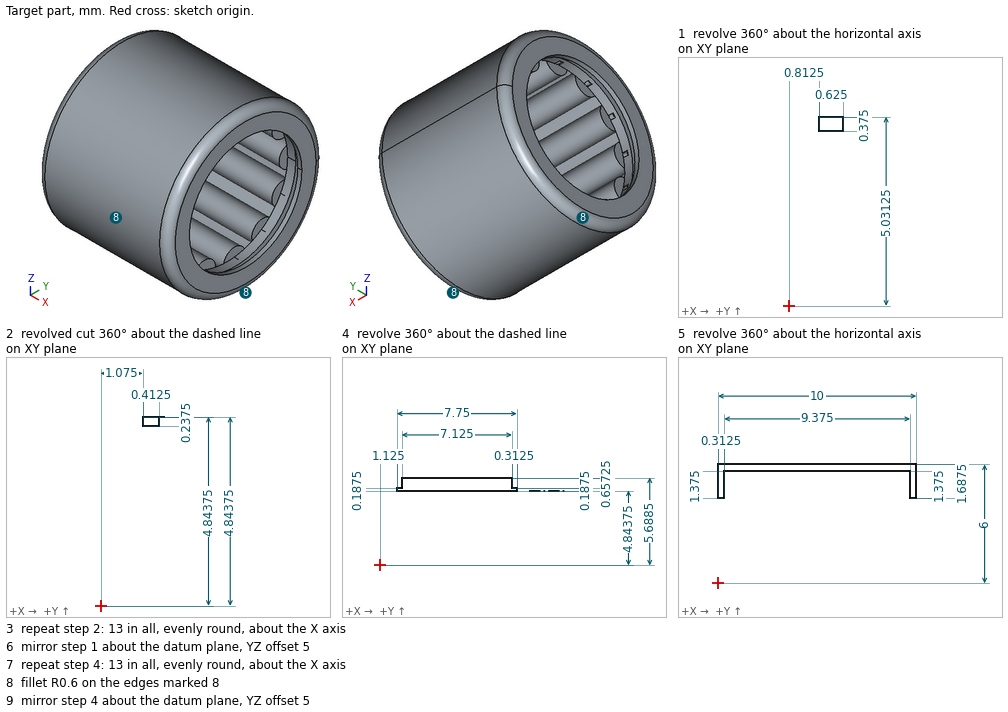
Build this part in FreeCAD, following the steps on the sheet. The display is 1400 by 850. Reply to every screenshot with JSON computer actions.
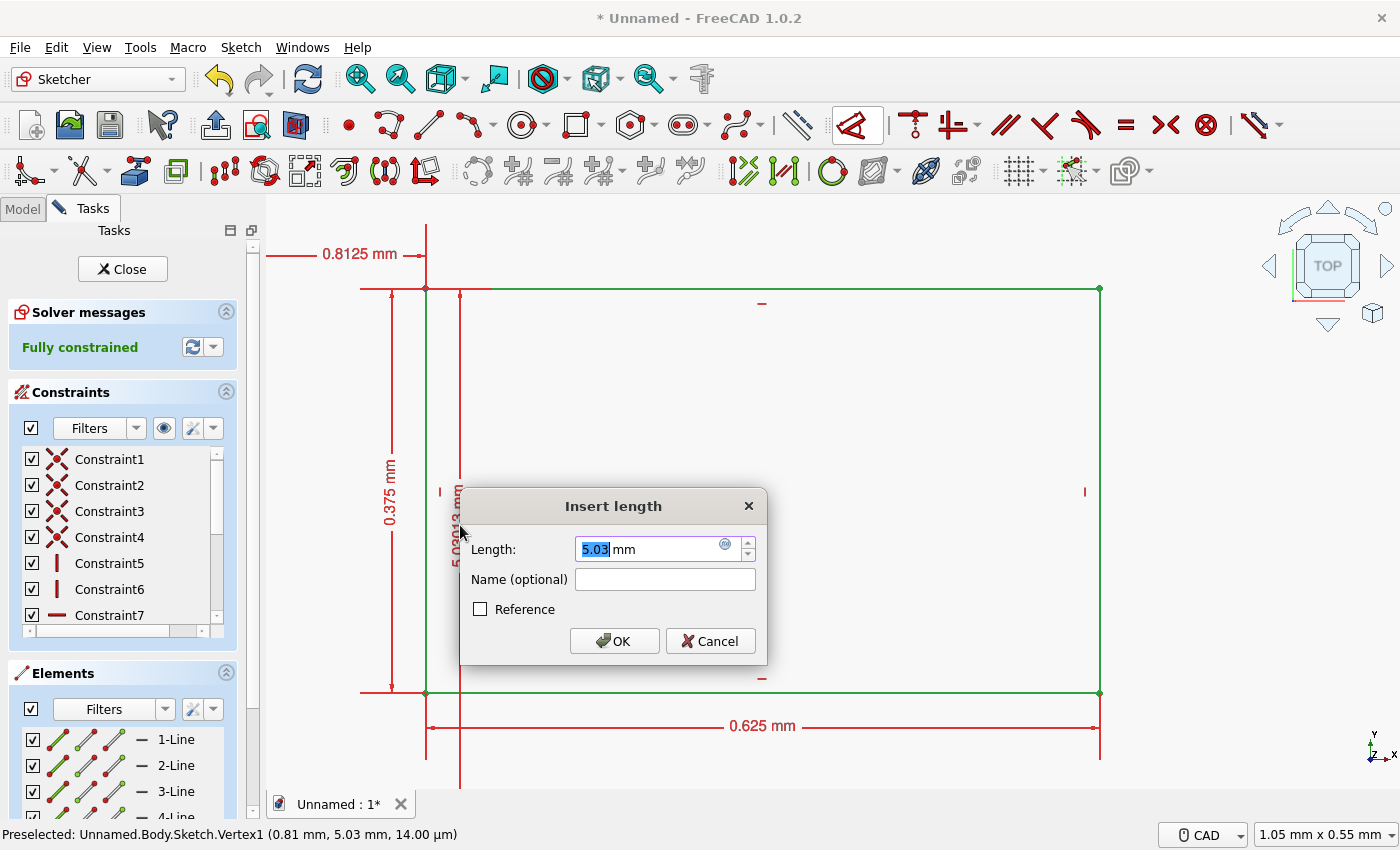
{"action": "type", "text": "5.03125"}
{"action": "key", "text": "Return"}
{"action": "key", "text": "Escape"}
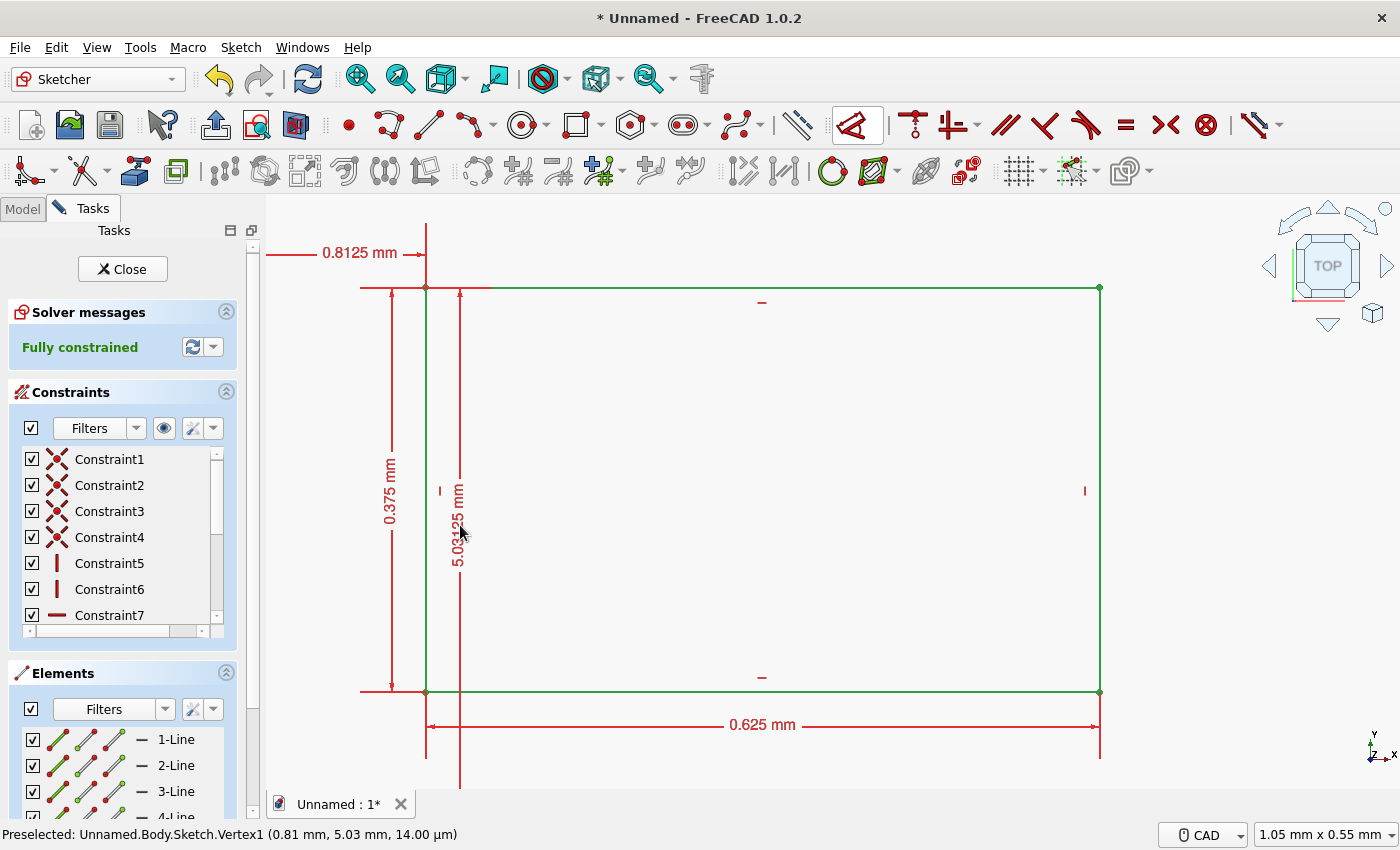
{"action": "left_click", "coordinate": [123, 269]}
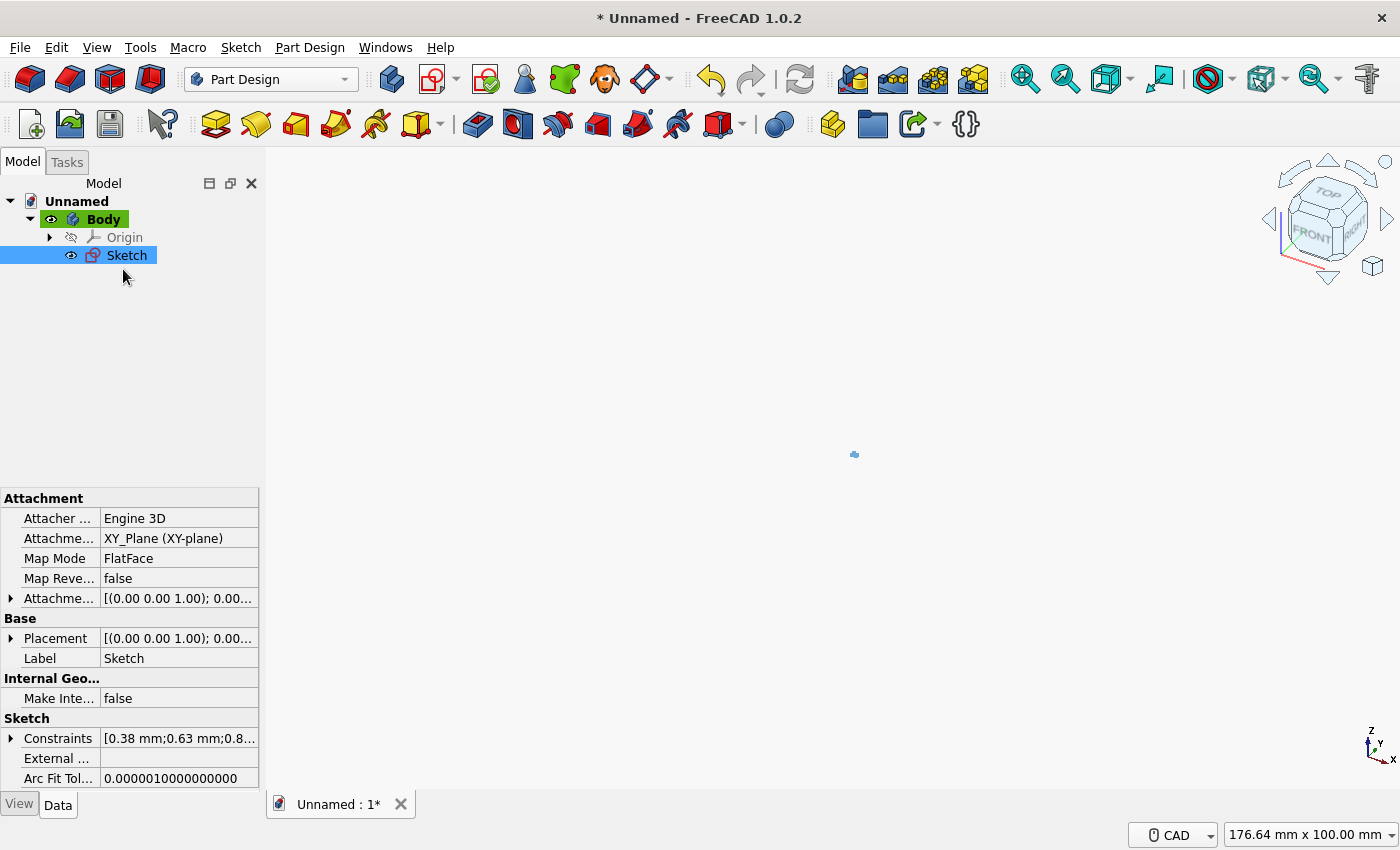
{"action": "left_click", "coordinate": [256, 124]}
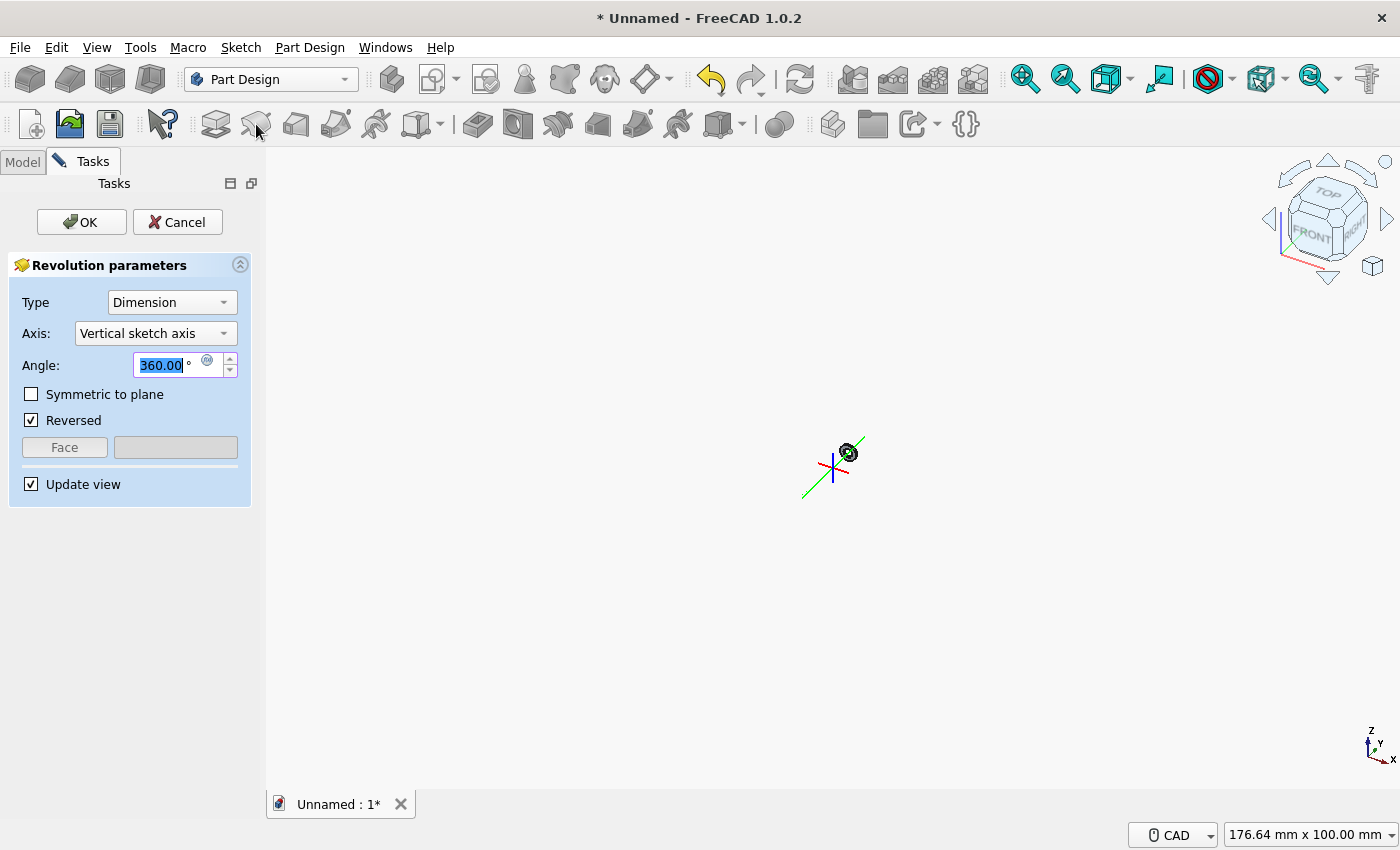
{"action": "left_click", "coordinate": [156, 334]}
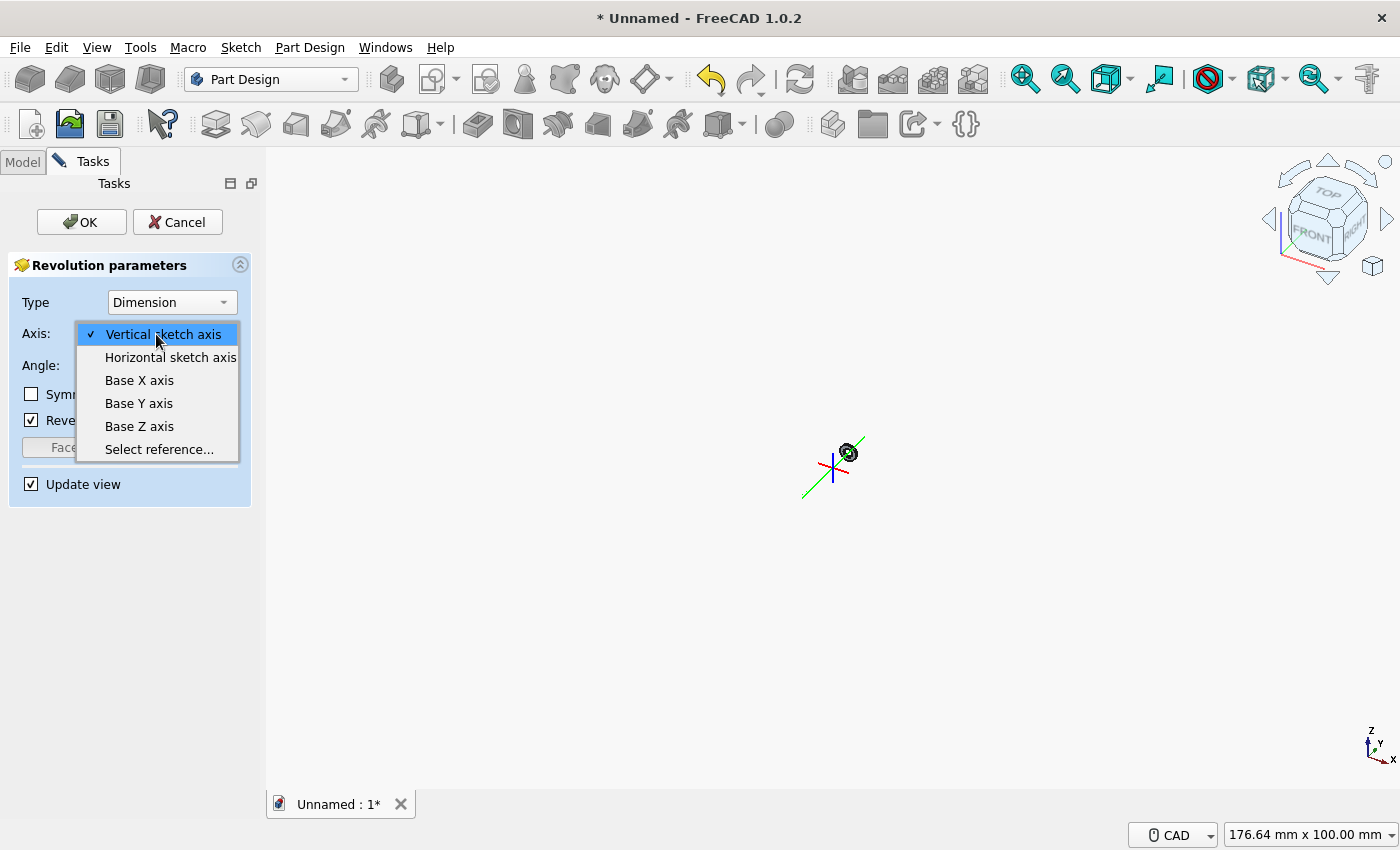
{"action": "left_click", "coordinate": [156, 358]}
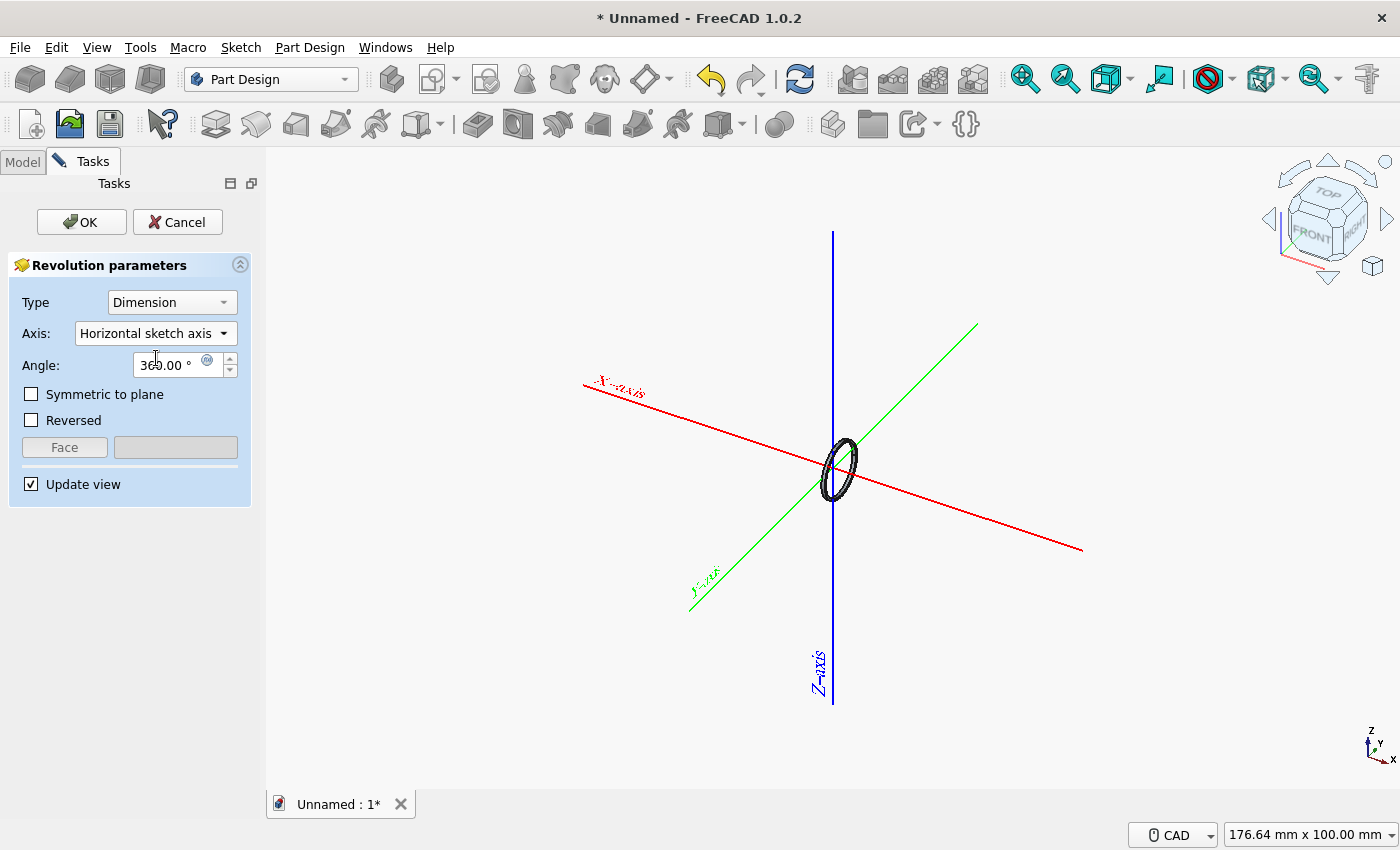
{"action": "left_click", "coordinate": [82, 222]}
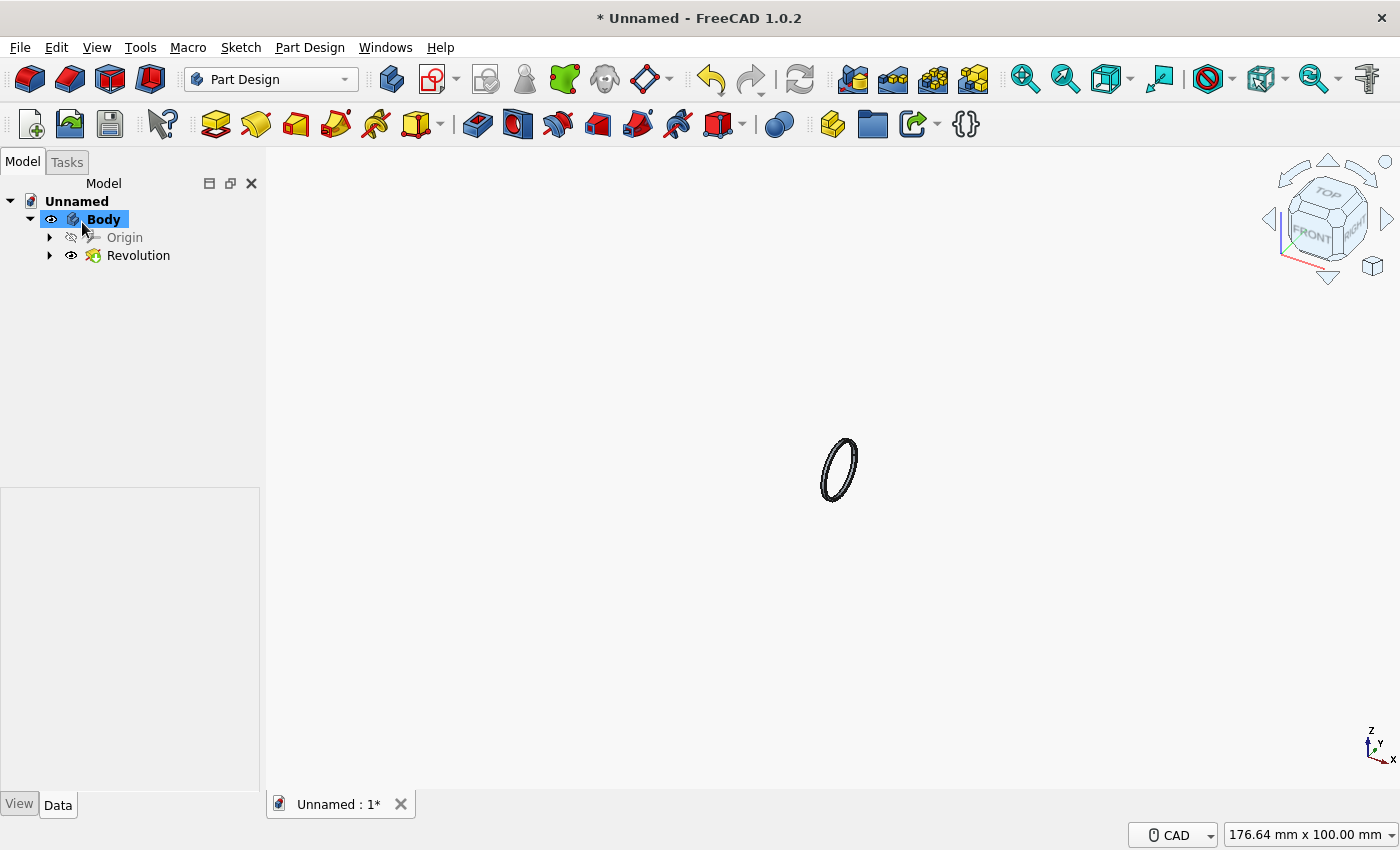
{"action": "left_click", "coordinate": [1026, 80]}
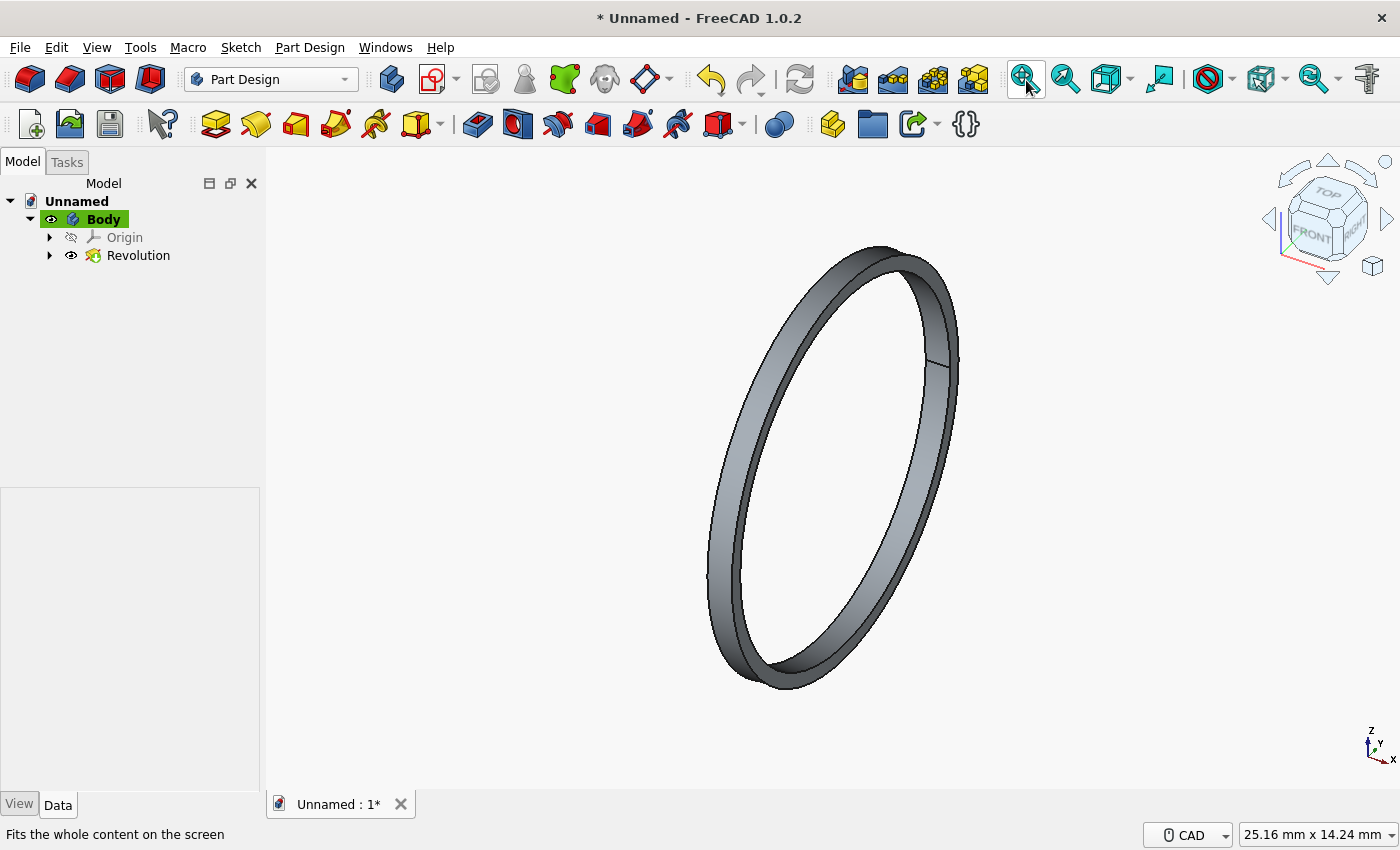
{"action": "left_click", "coordinate": [432, 80]}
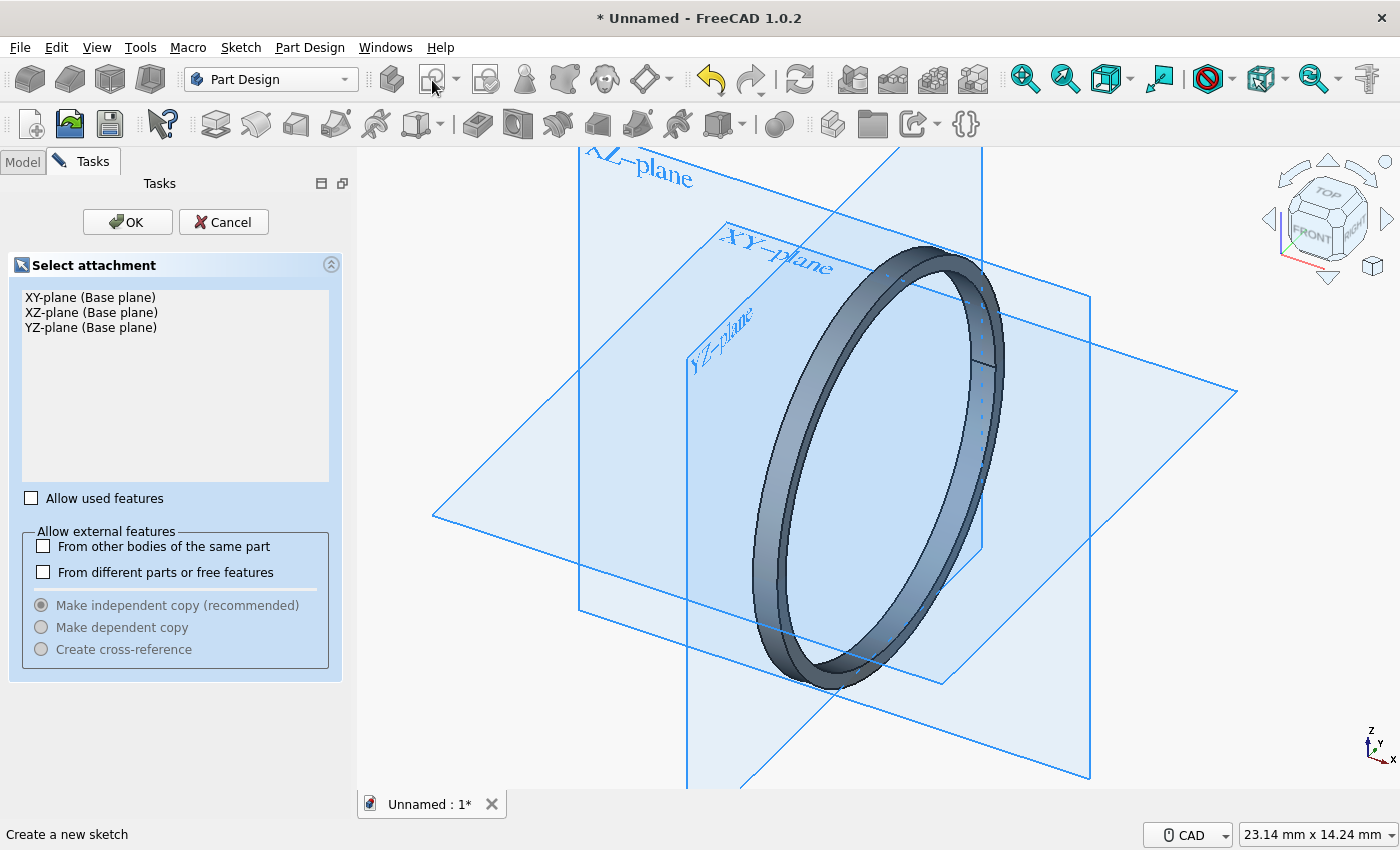
{"action": "left_click", "coordinate": [82, 298]}